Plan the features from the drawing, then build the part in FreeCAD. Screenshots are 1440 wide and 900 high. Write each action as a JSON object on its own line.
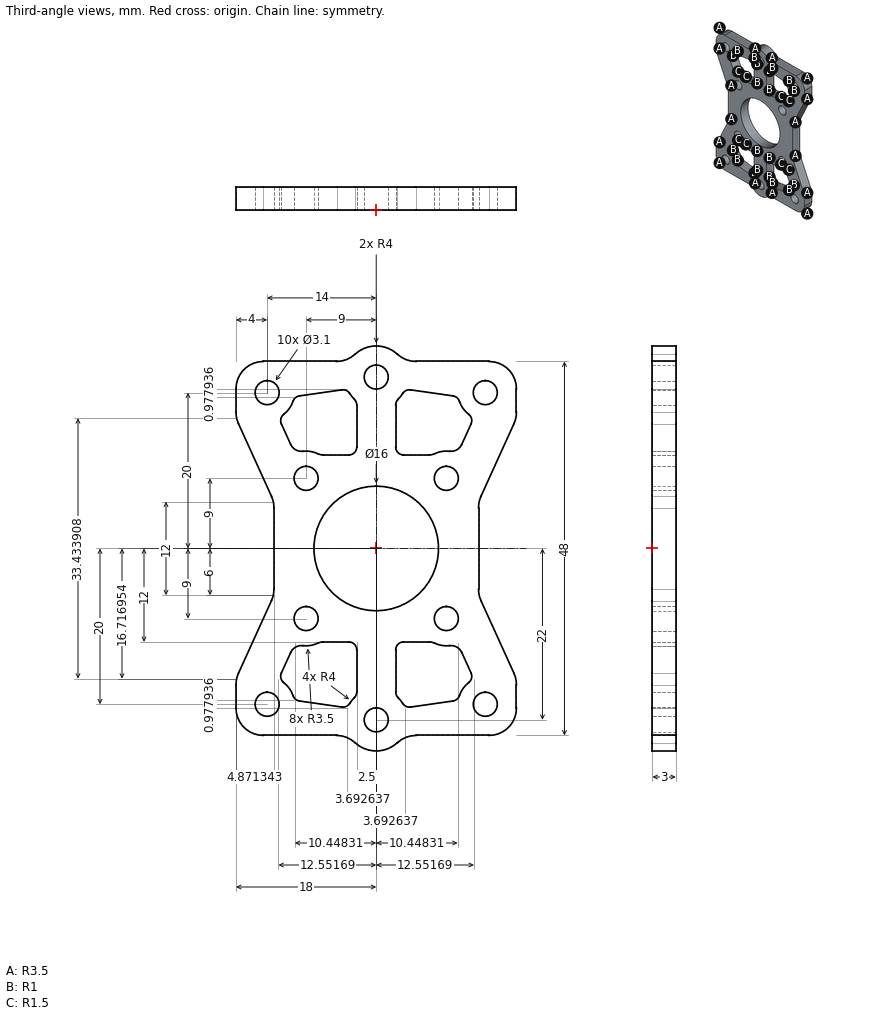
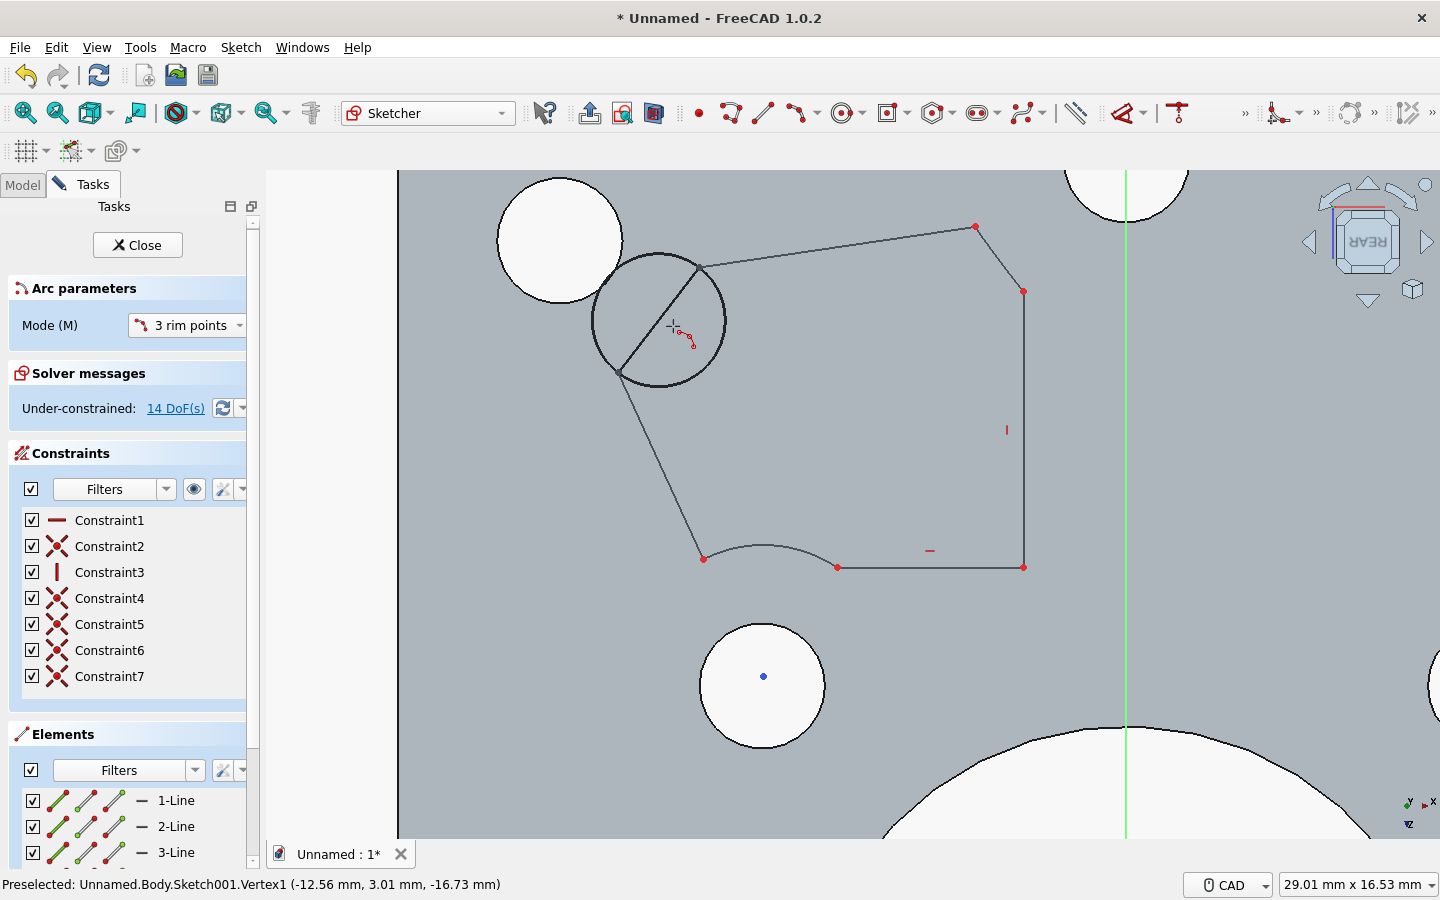
{"action": "left_click", "coordinate": [673, 326]}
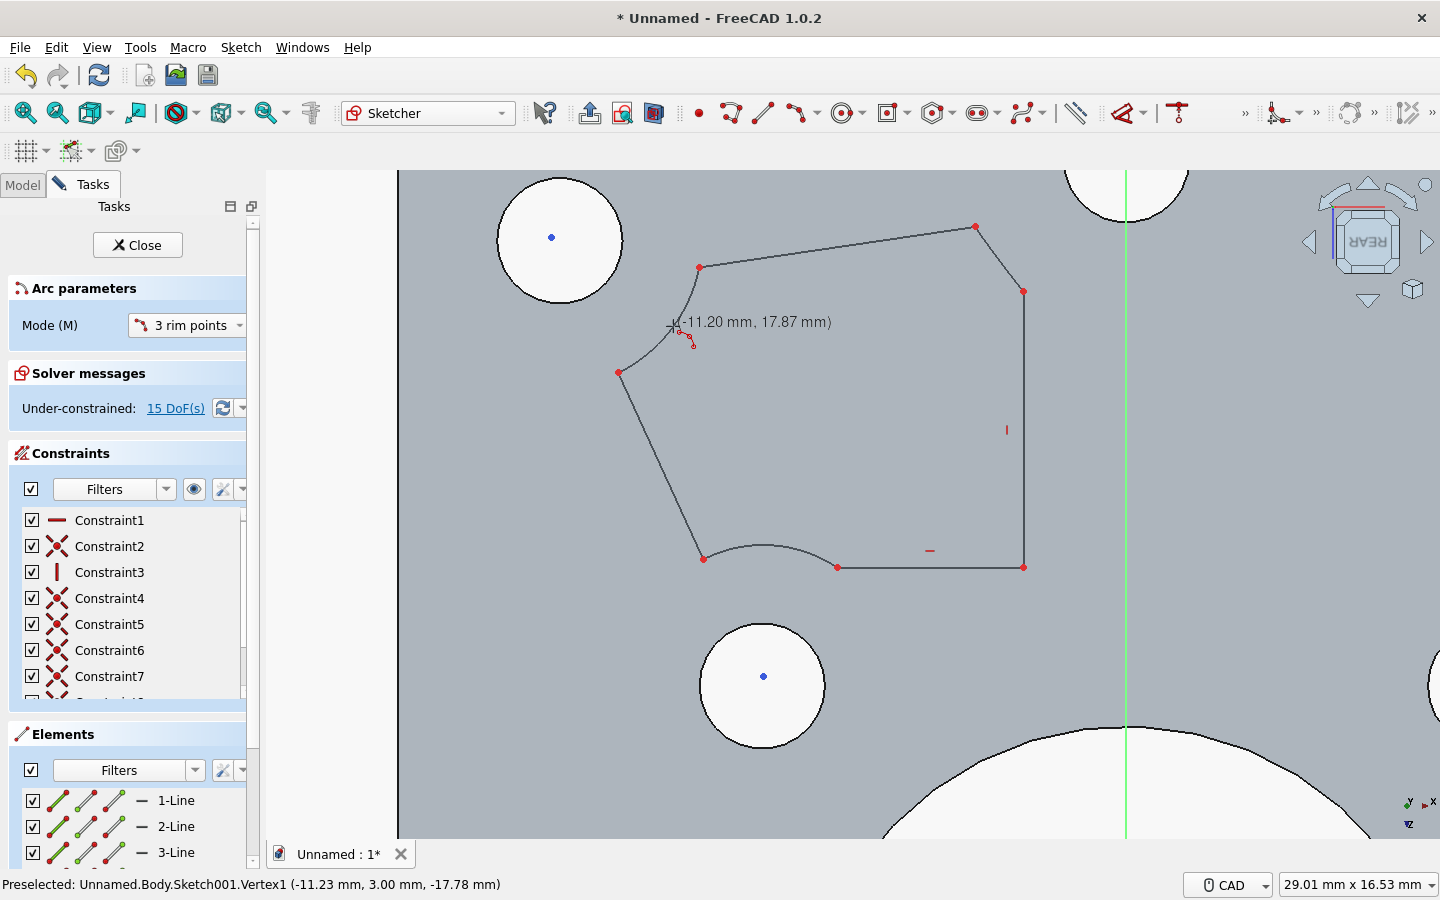
{"action": "left_click", "coordinate": [732, 114]}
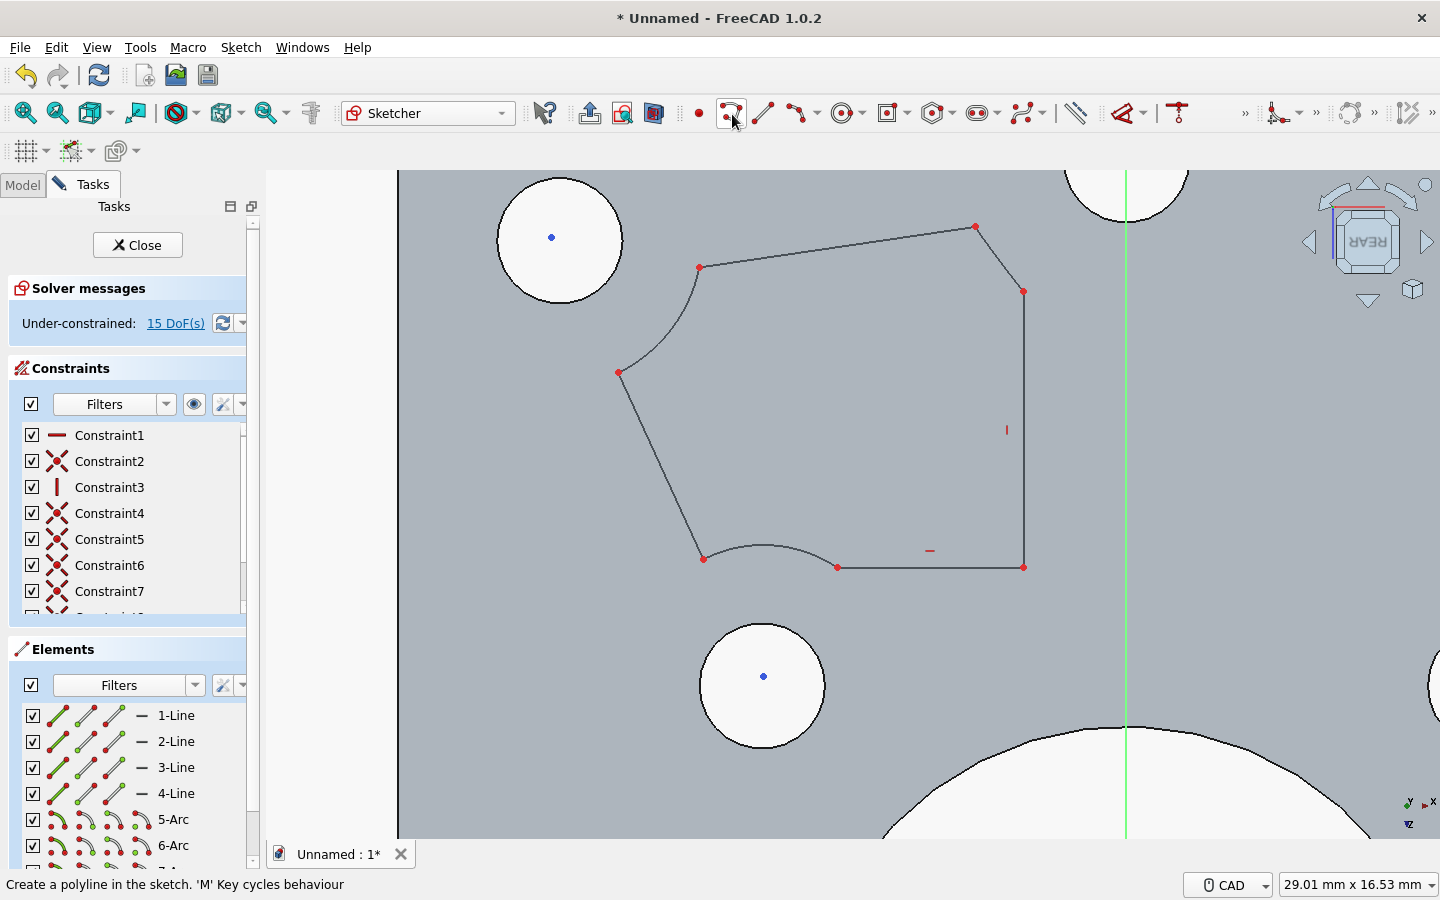
{"action": "scroll", "coordinate": [673, 326], "scroll_direction": "down", "scroll_amount": 7}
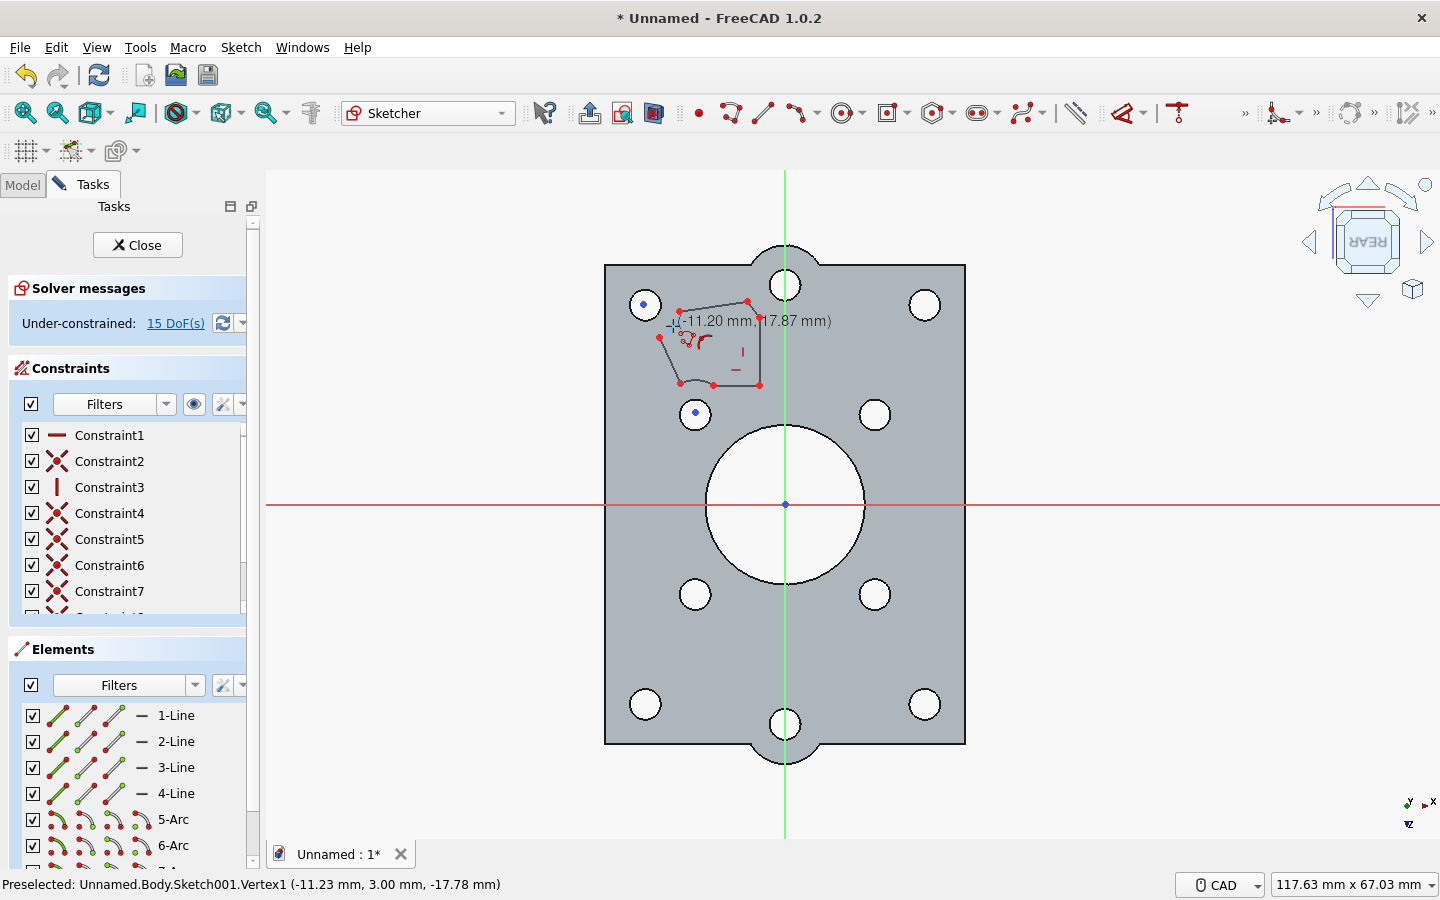
{"action": "left_click", "coordinate": [810, 316]}
{"action": "left_click", "coordinate": [810, 385]}
{"action": "left_click", "coordinate": [857, 385]}
{"action": "right_click", "coordinate": [857, 385]}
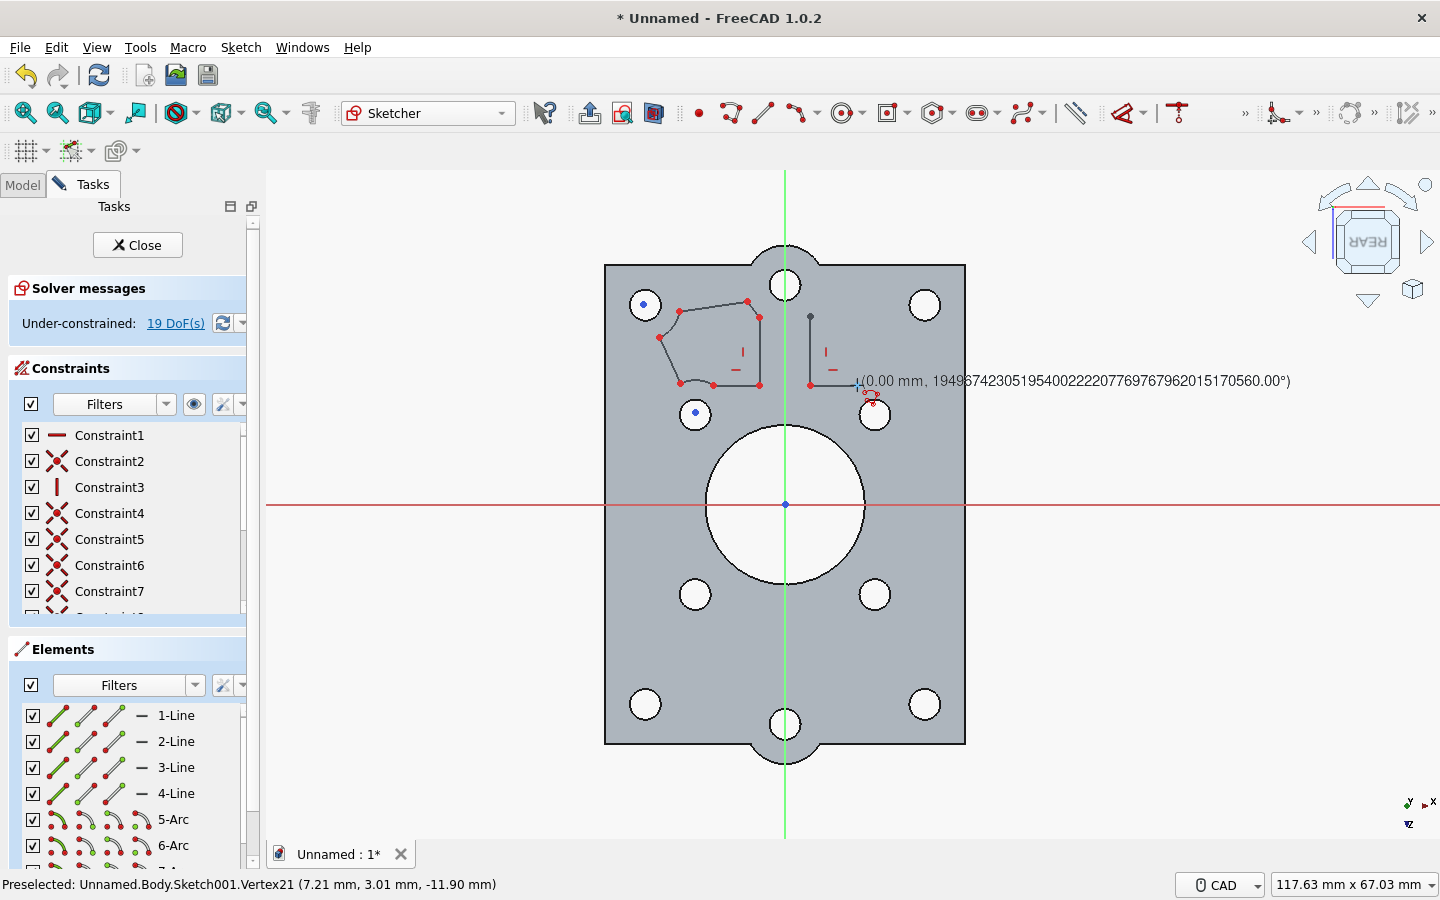
{"action": "left_click", "coordinate": [764, 114]}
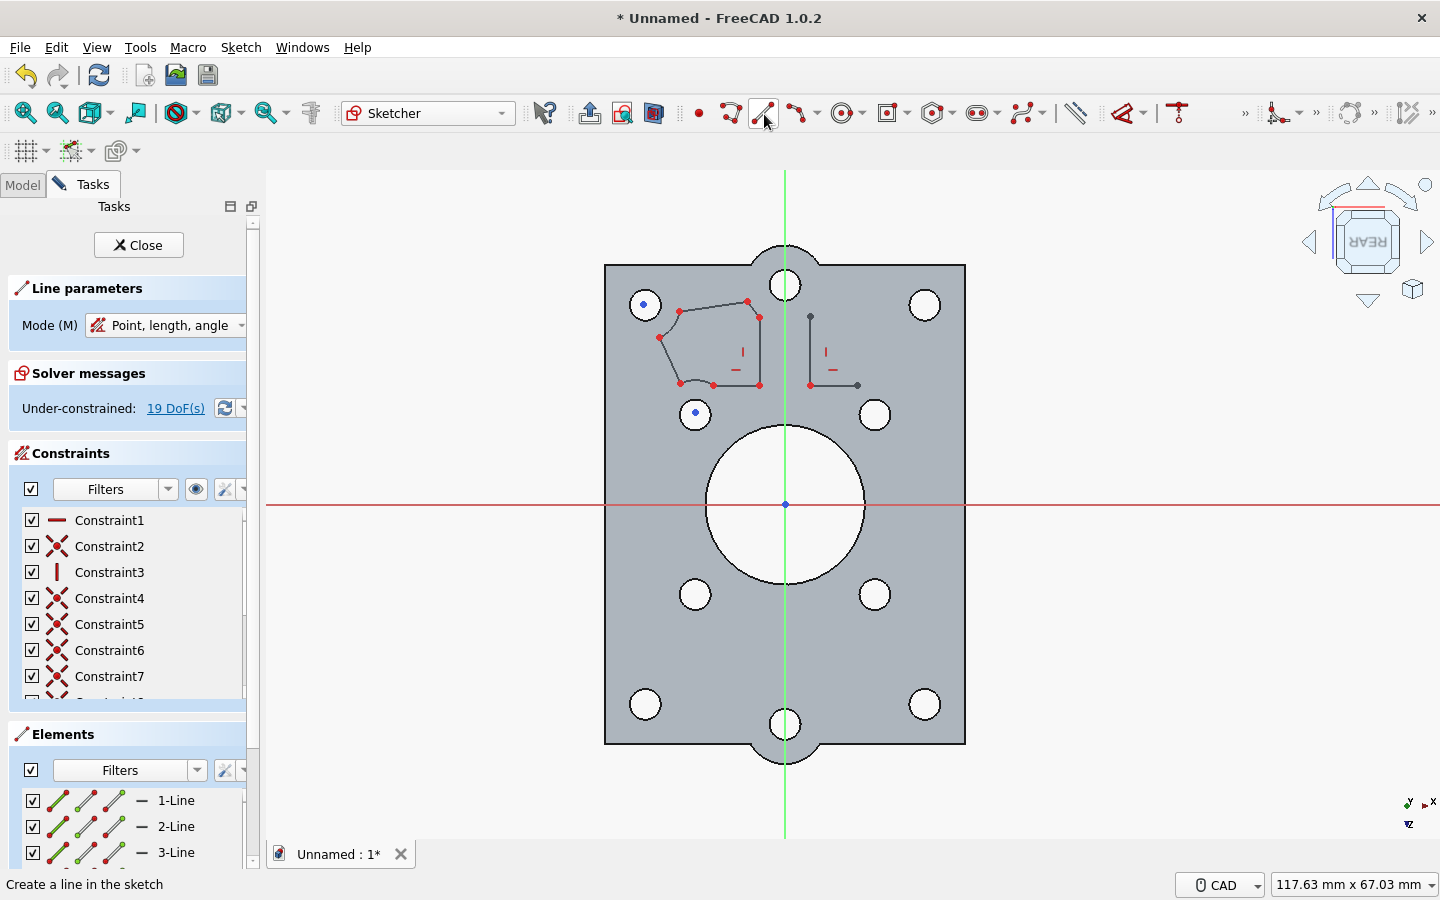
{"action": "left_click", "coordinate": [889, 383]}
{"action": "left_click", "coordinate": [910, 337]}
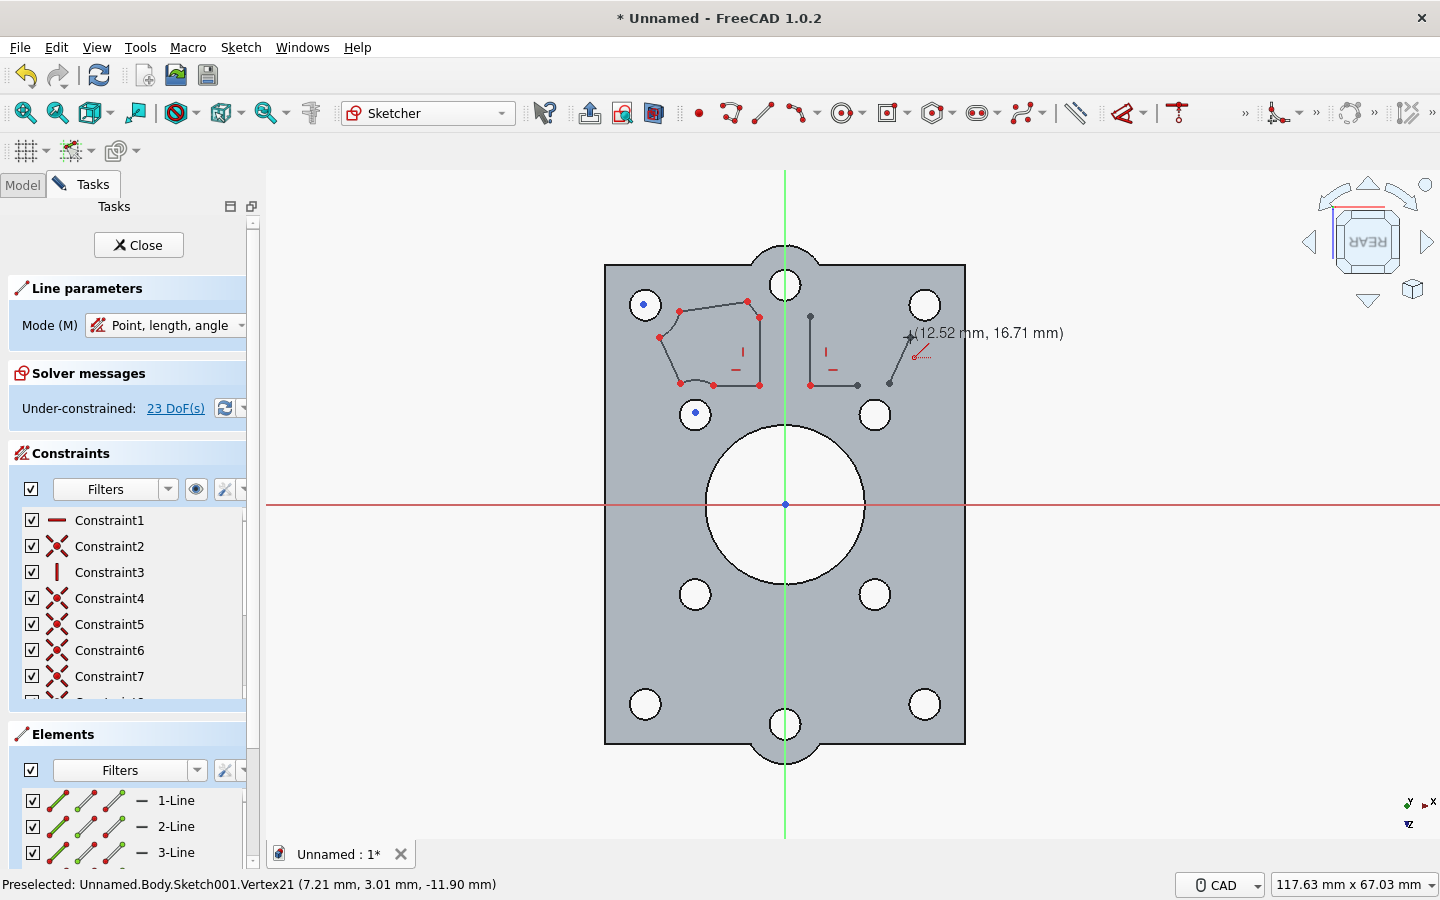
{"action": "left_click", "coordinate": [890, 310]}
{"action": "left_click", "coordinate": [822, 301]}